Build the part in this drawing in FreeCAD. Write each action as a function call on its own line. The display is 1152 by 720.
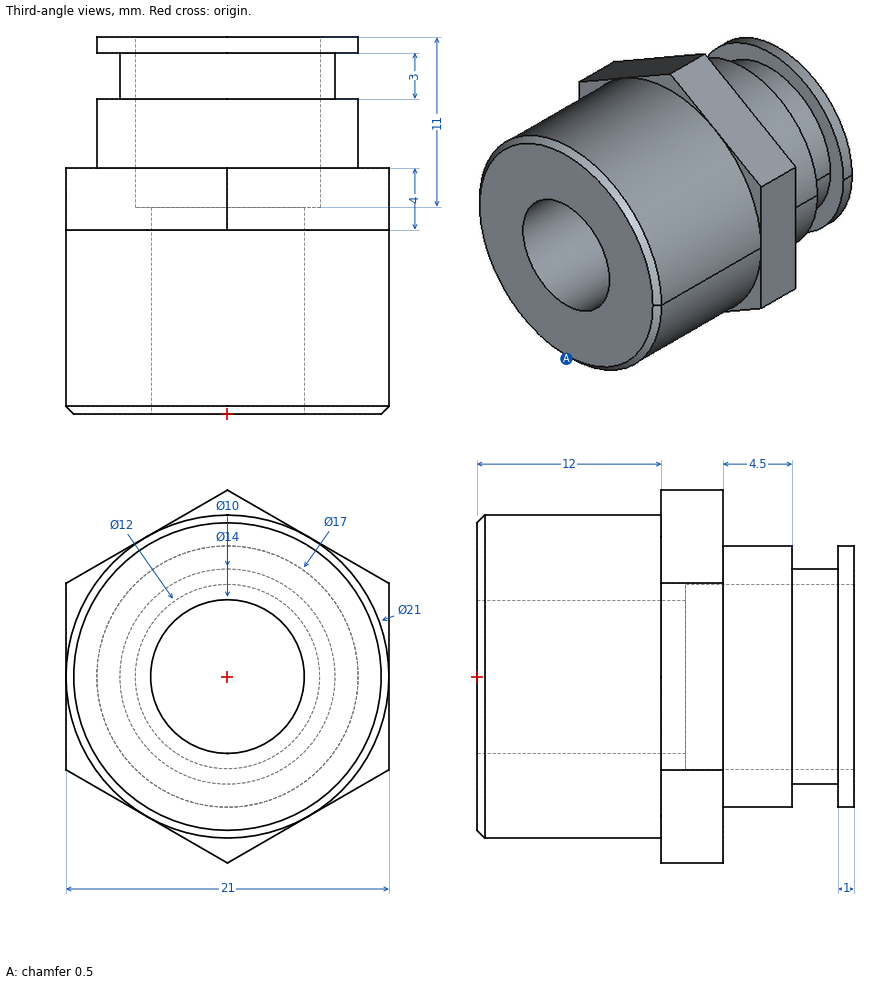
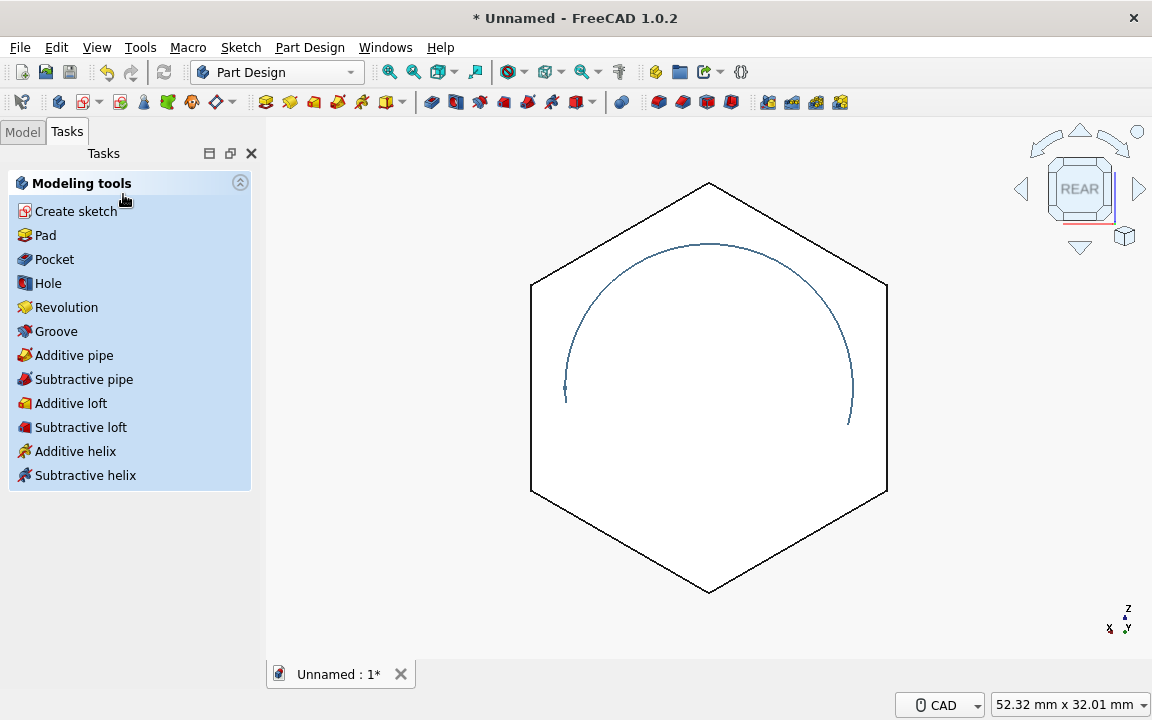
click(266, 102)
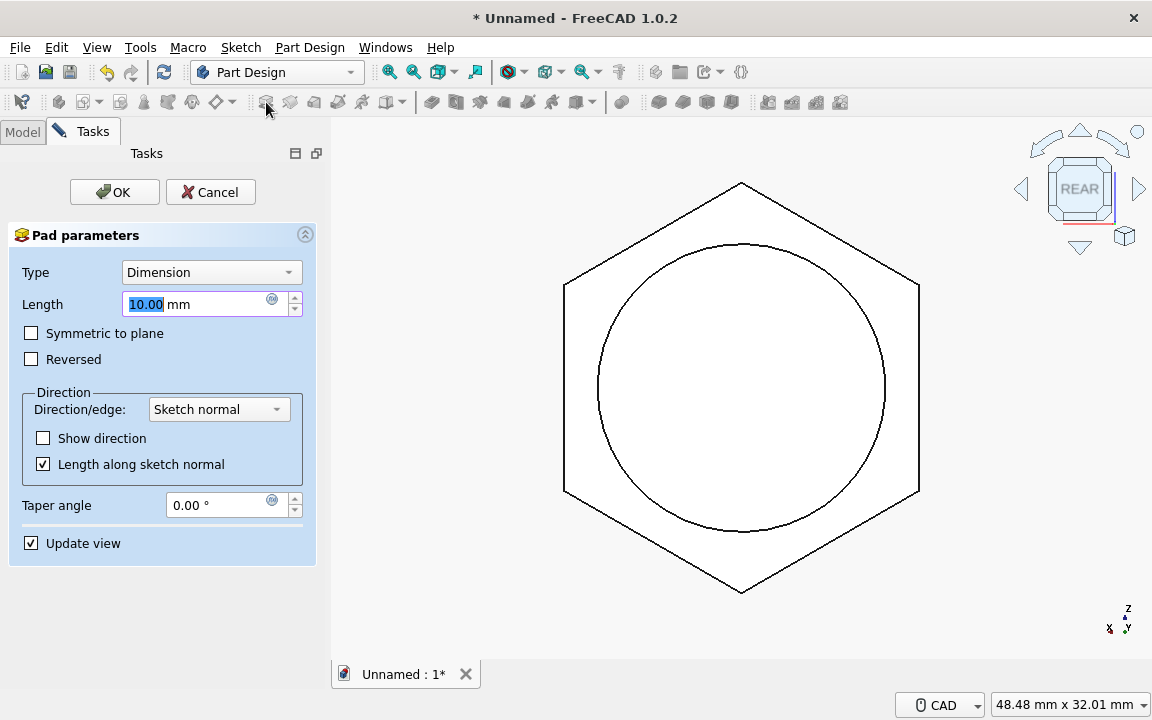
text(4.5)
key(Tab)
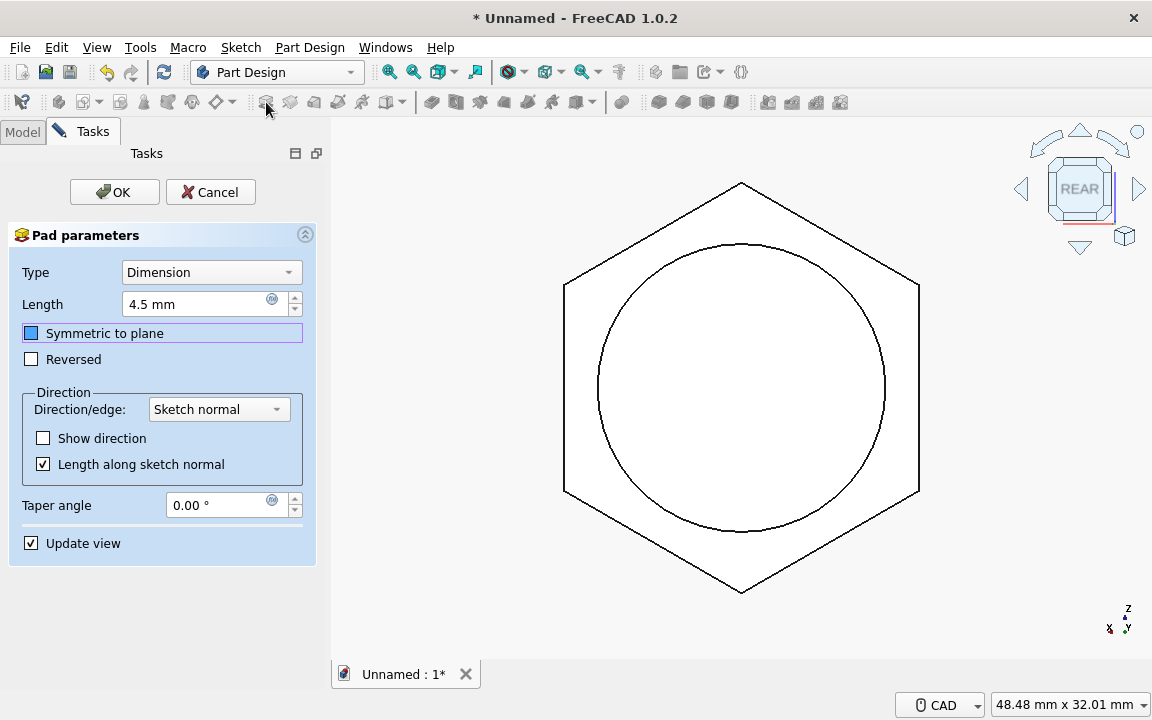
click(115, 192)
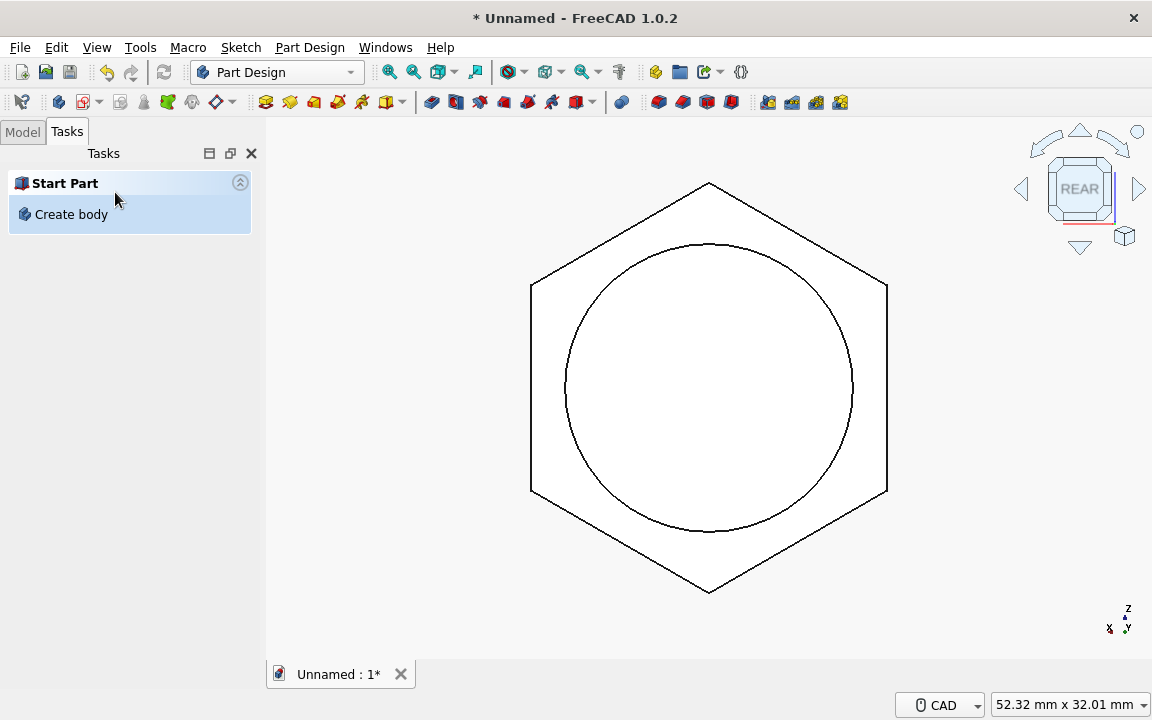
click(709, 387)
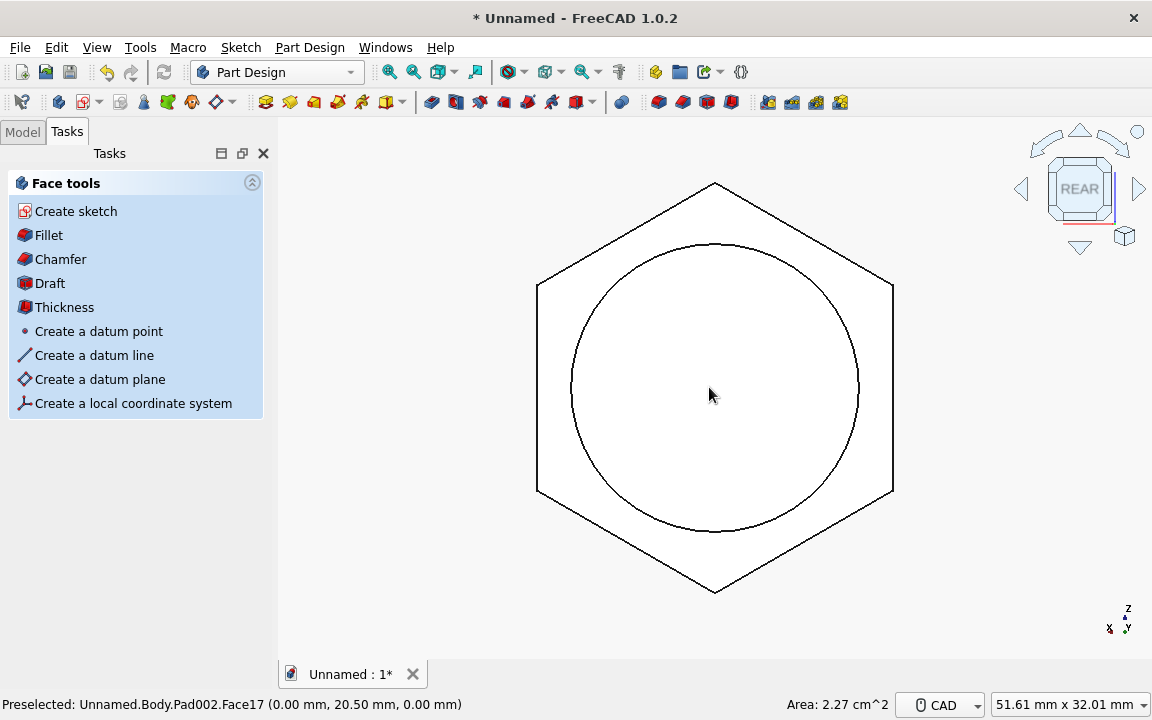
click(84, 102)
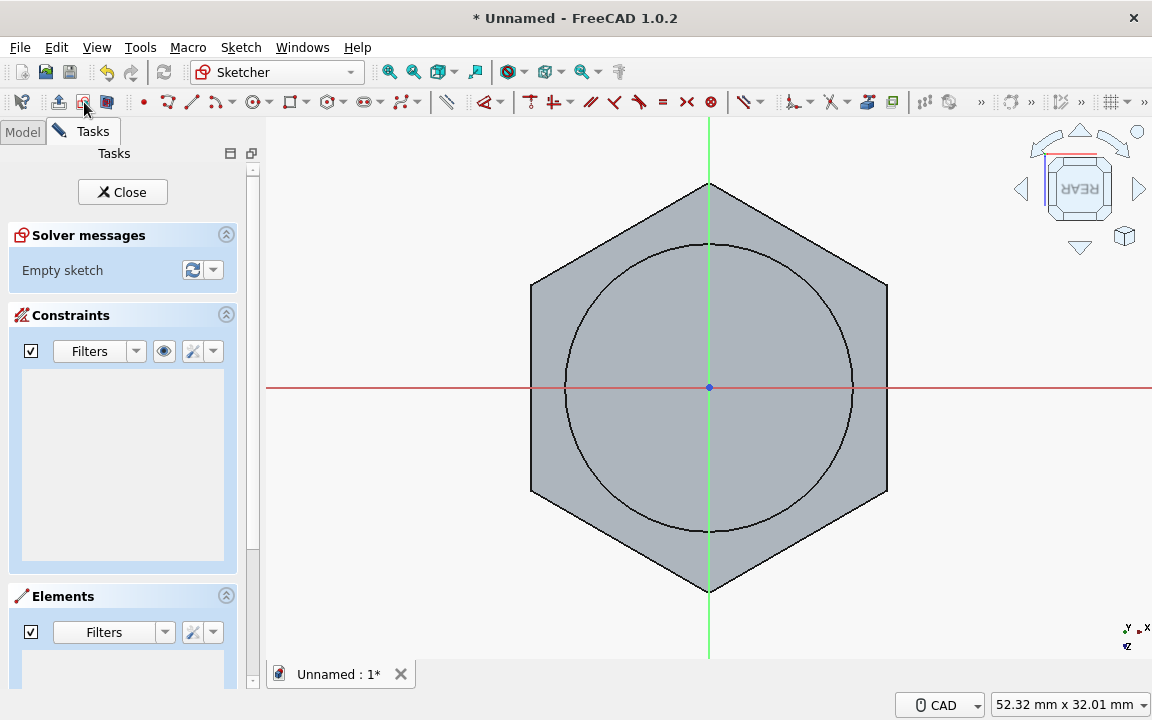
scroll(848, 388, up, 2)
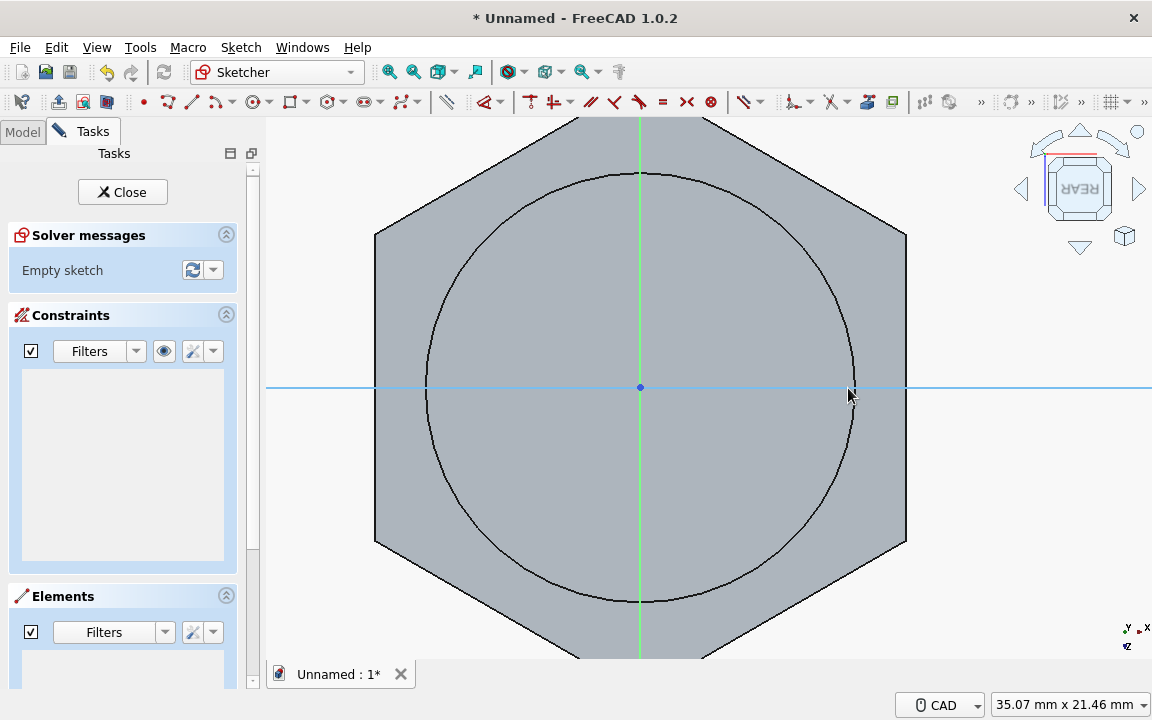
key(g)
key(c)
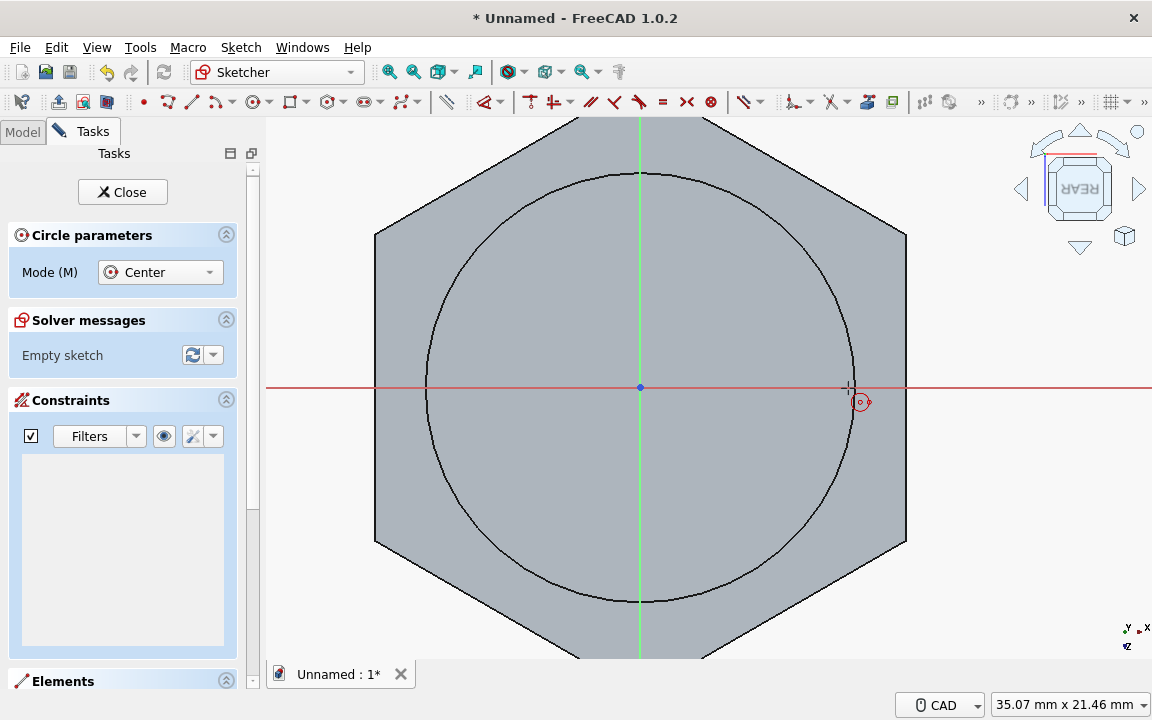
click(640, 388)
move(765, 263)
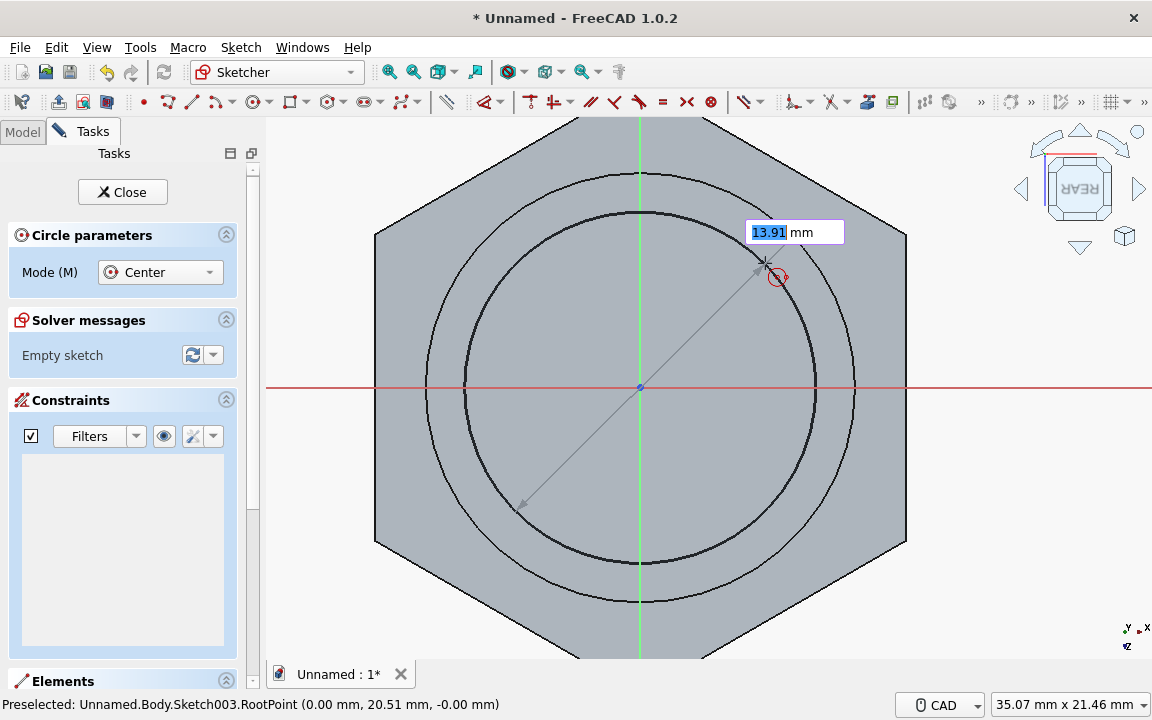
text(14)
key(Return)
key(Escape)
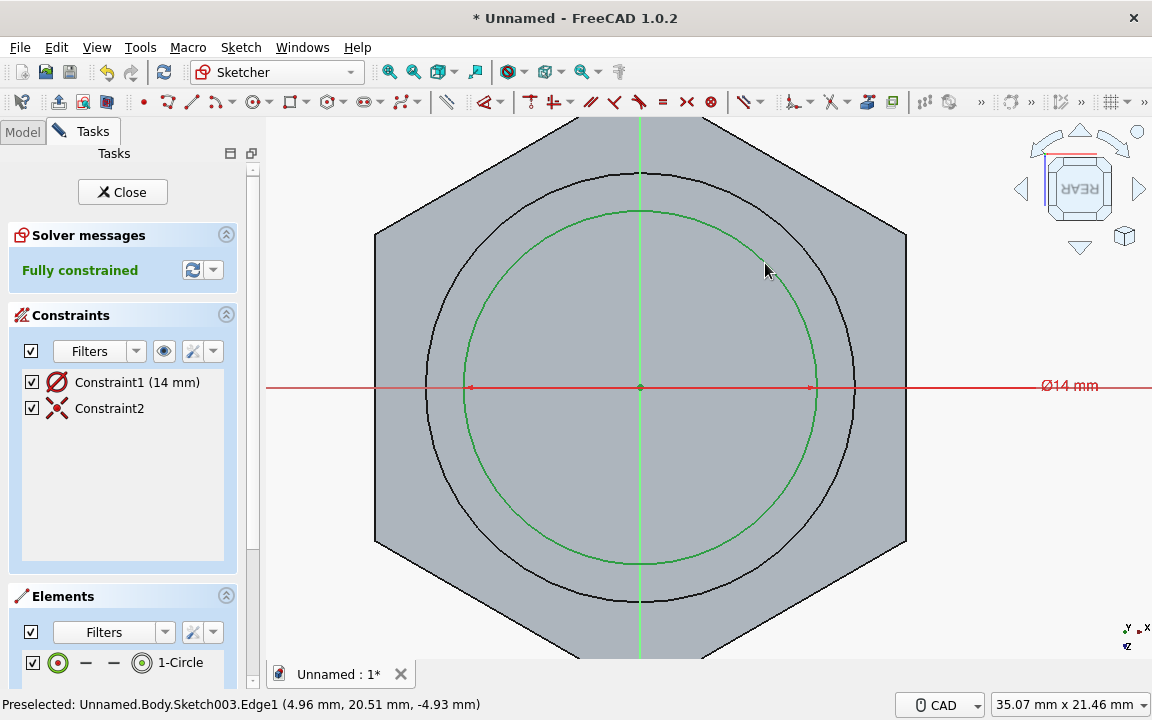
click(123, 192)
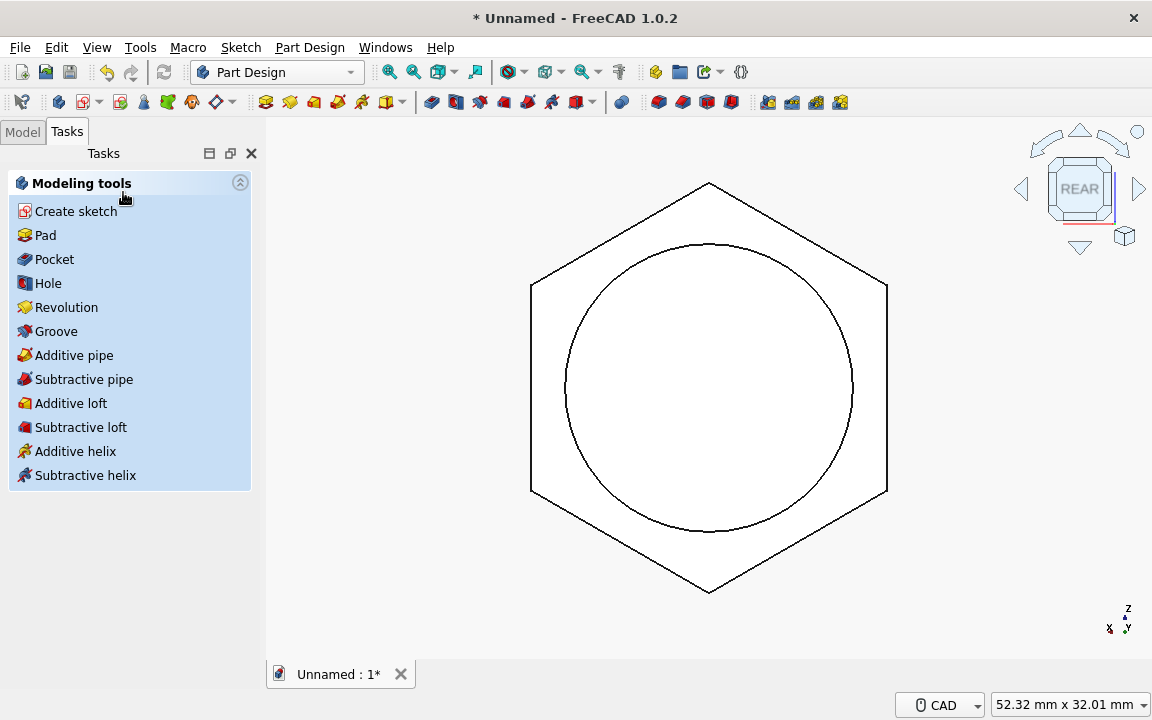
click(266, 102)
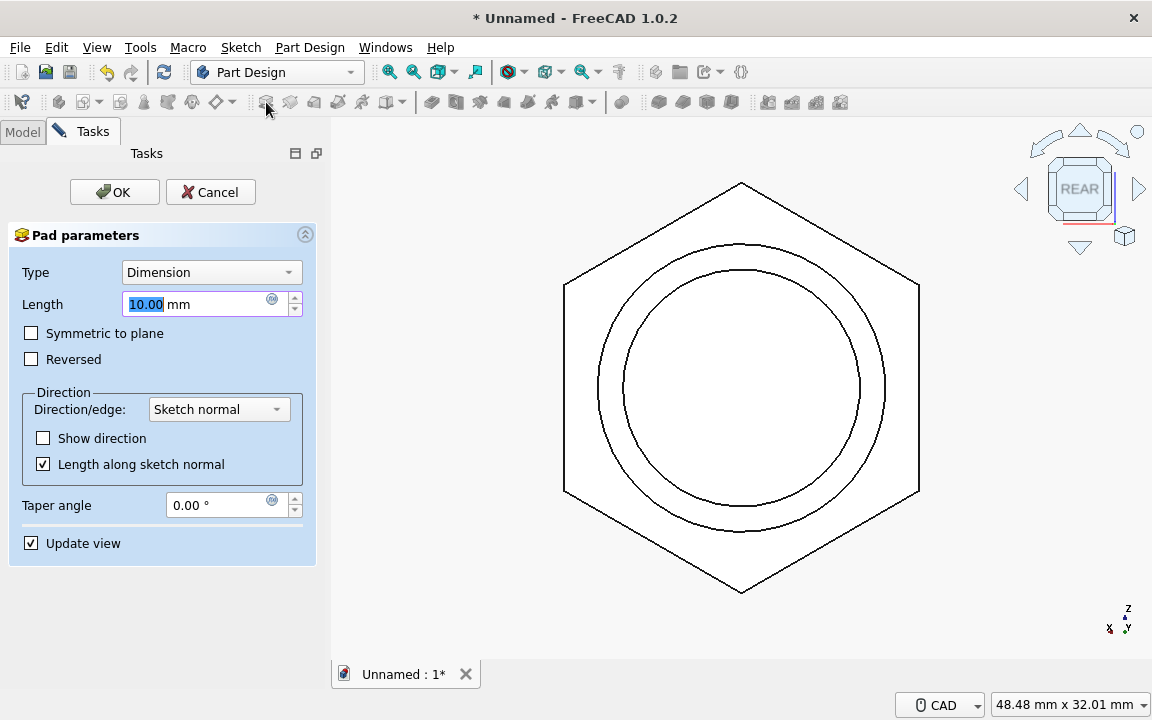
text(3)
key(Tab)